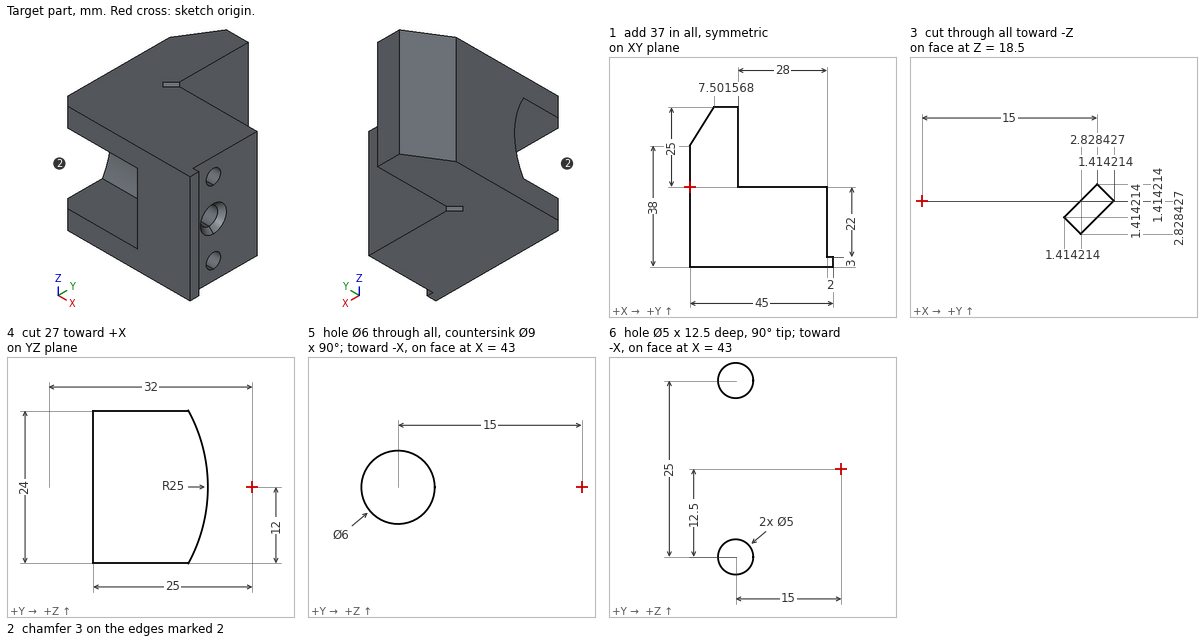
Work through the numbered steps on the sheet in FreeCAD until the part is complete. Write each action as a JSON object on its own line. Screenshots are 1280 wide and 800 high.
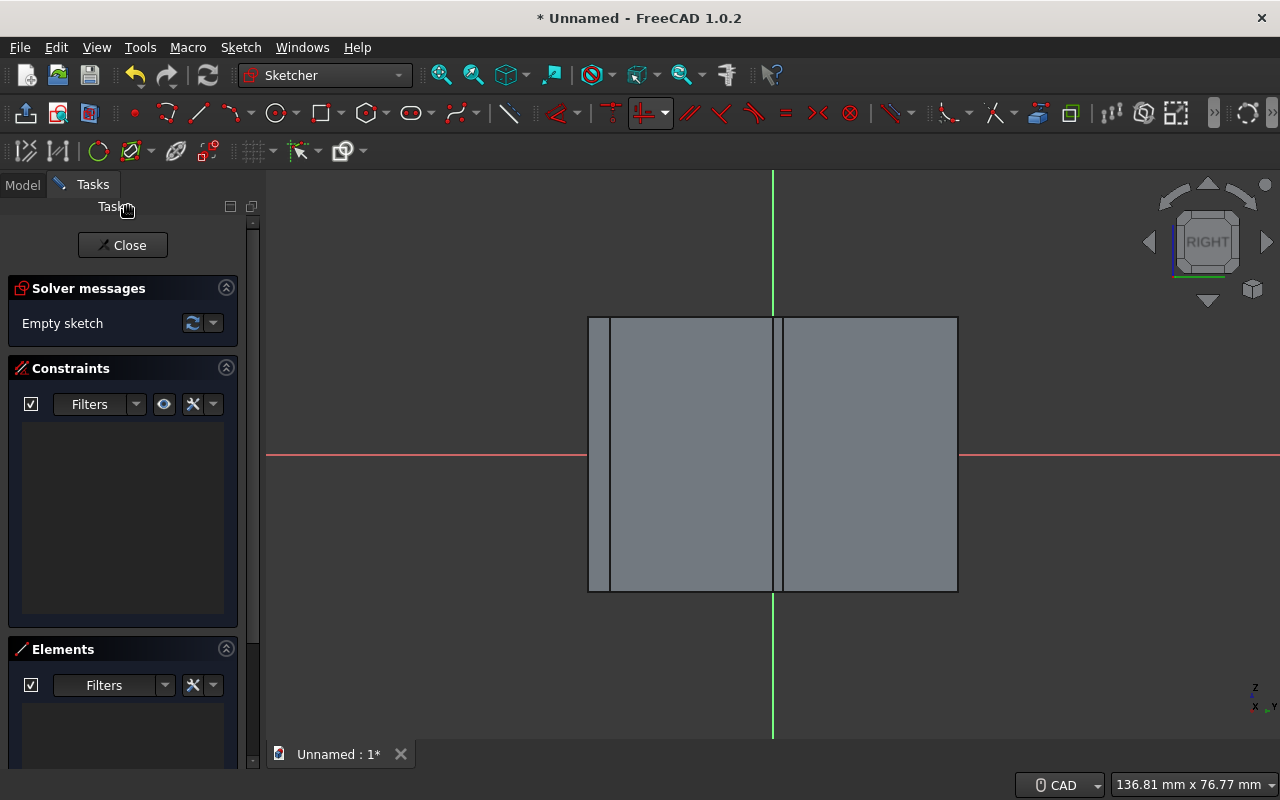
{"action": "left_click", "coordinate": [90, 114]}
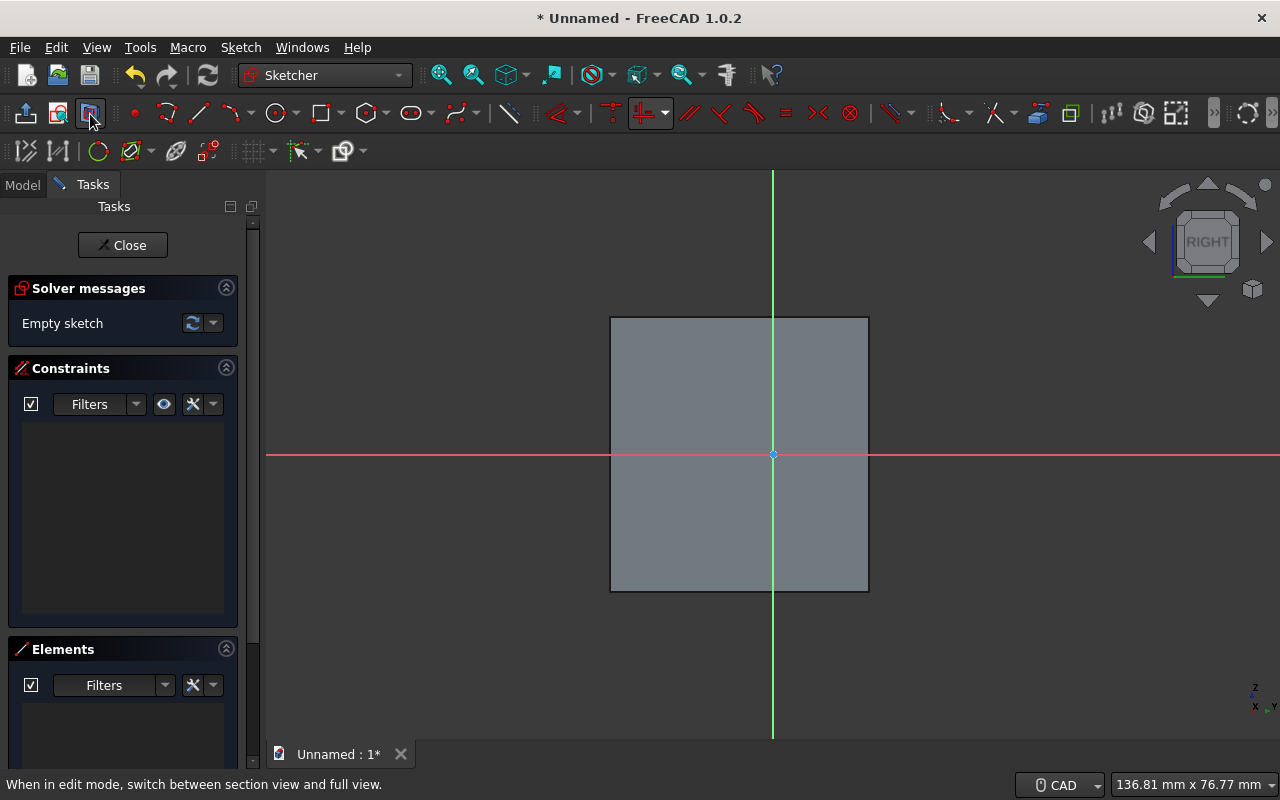
{"action": "scroll", "coordinate": [661, 454], "scroll_direction": "up", "scroll_amount": 4}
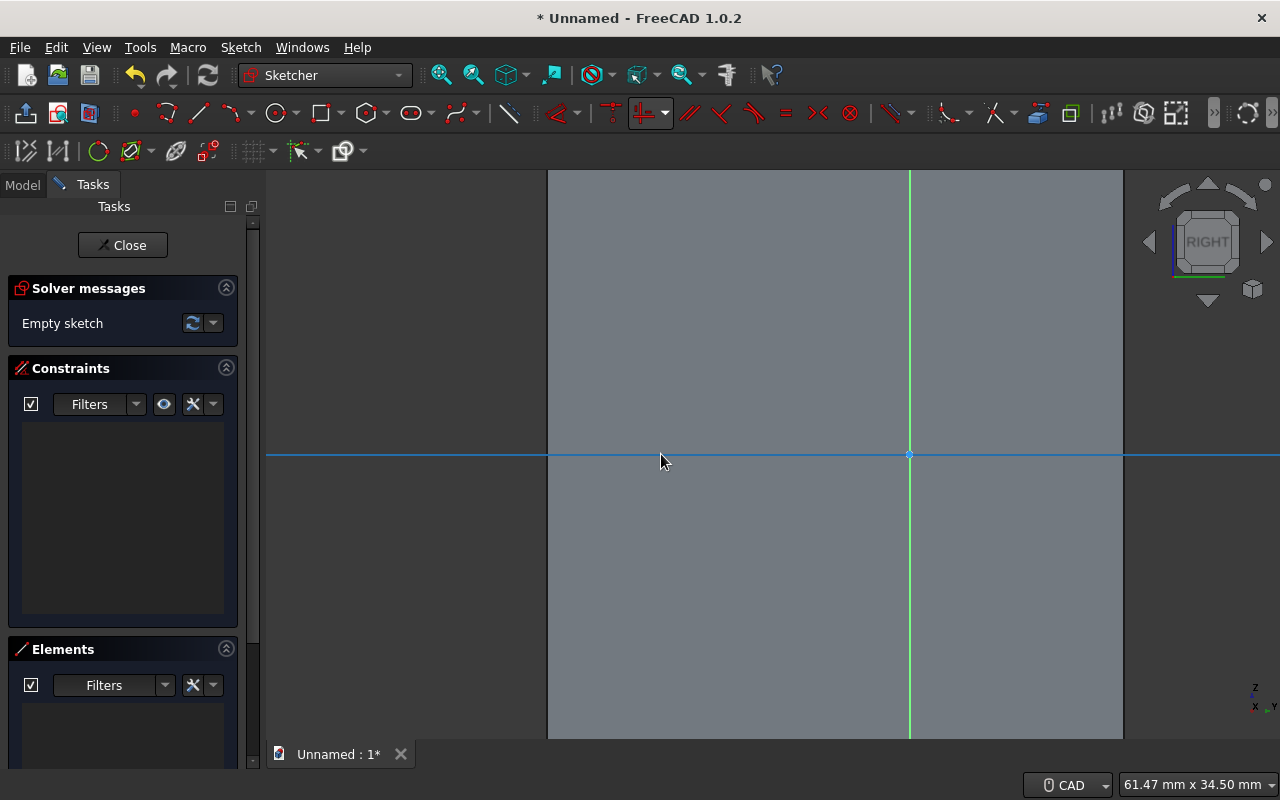
{"action": "left_click", "coordinate": [168, 114]}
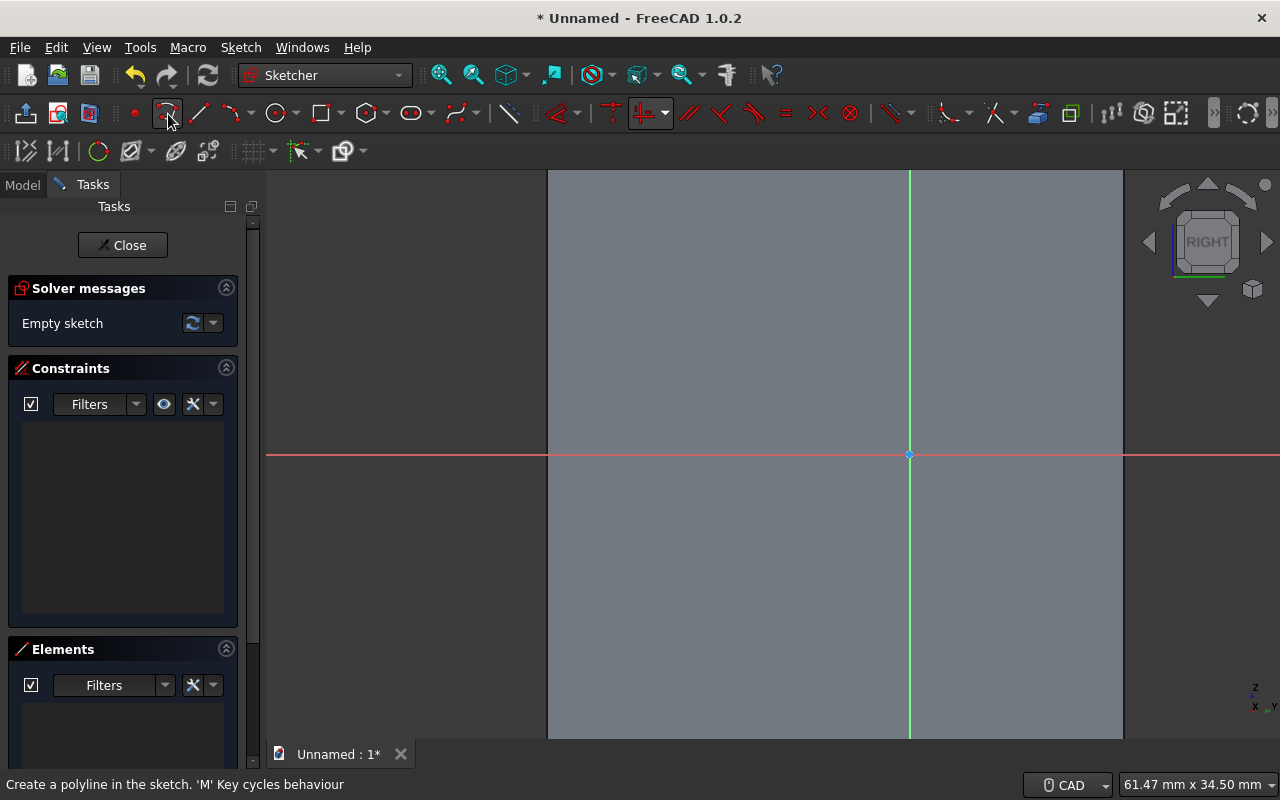
{"action": "left_click", "coordinate": [744, 652]}
{"action": "left_click", "coordinate": [497, 652]}
{"action": "left_click", "coordinate": [497, 257]}
{"action": "left_click", "coordinate": [744, 257]}
{"action": "right_click", "coordinate": [744, 257]}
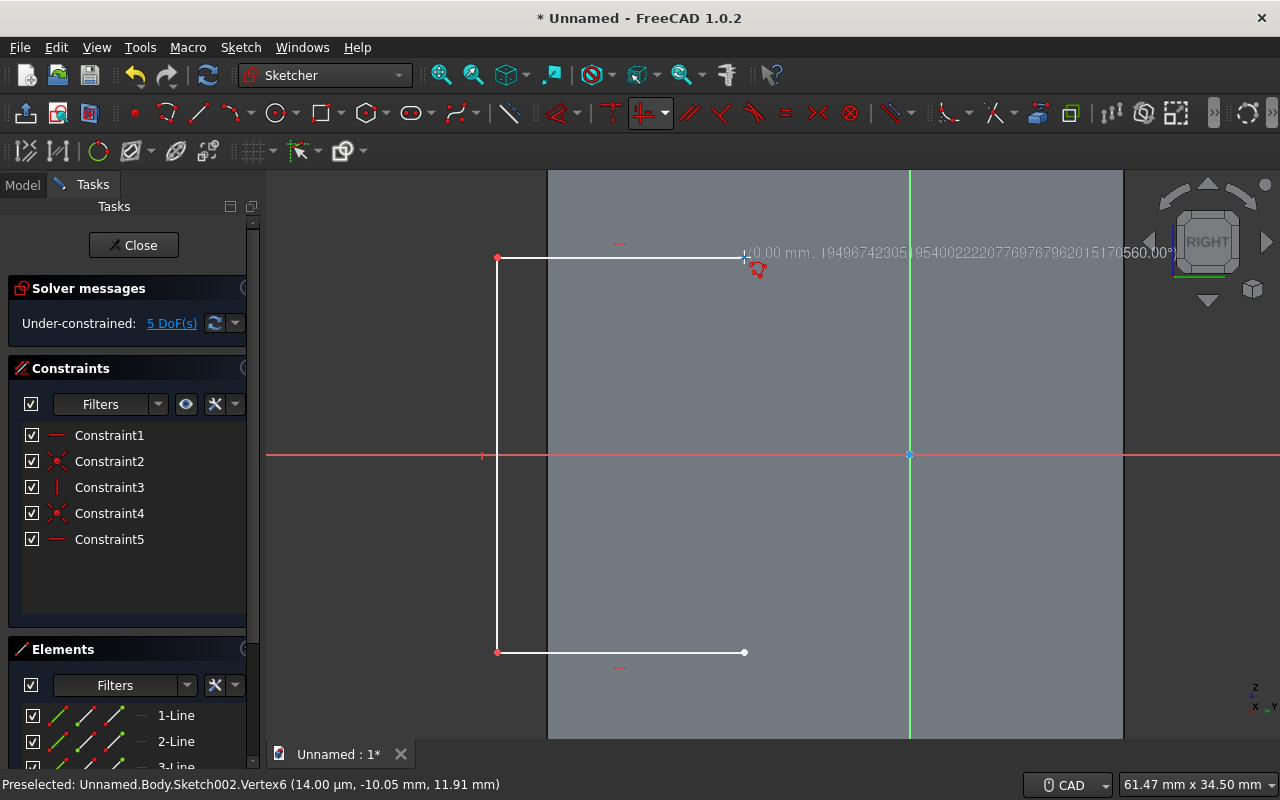
{"action": "left_click", "coordinate": [232, 114]}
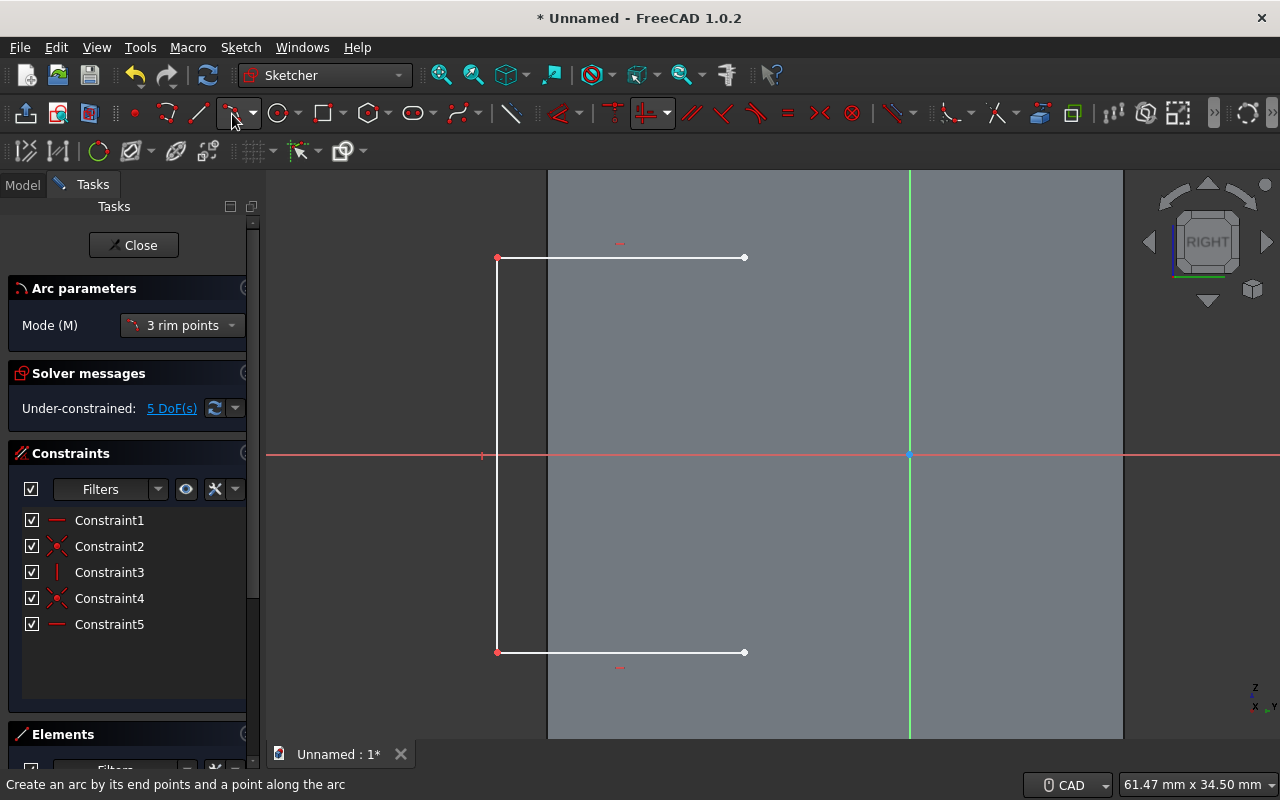
{"action": "left_click", "coordinate": [744, 258]}
{"action": "left_click", "coordinate": [744, 653]}
{"action": "left_click", "coordinate": [792, 496]}
{"action": "key", "text": "Escape"}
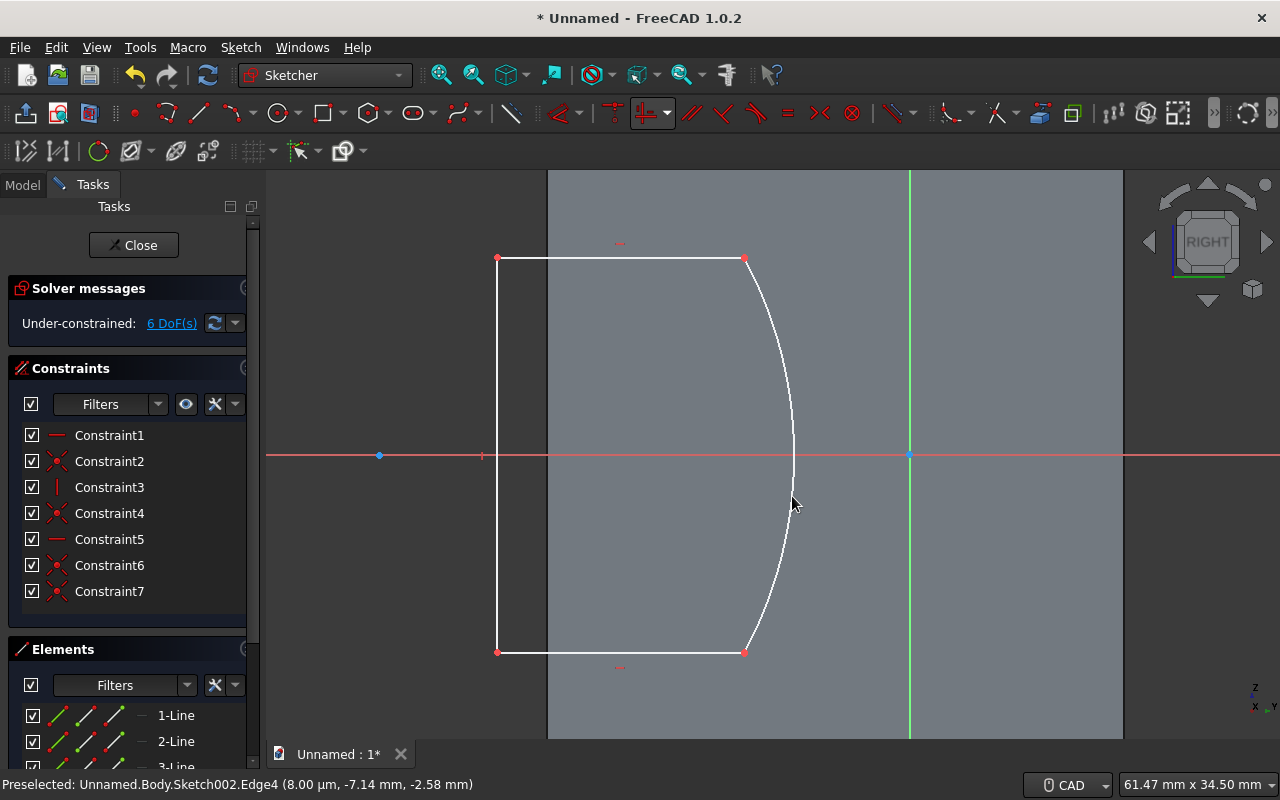
{"action": "left_click", "coordinate": [380, 456]}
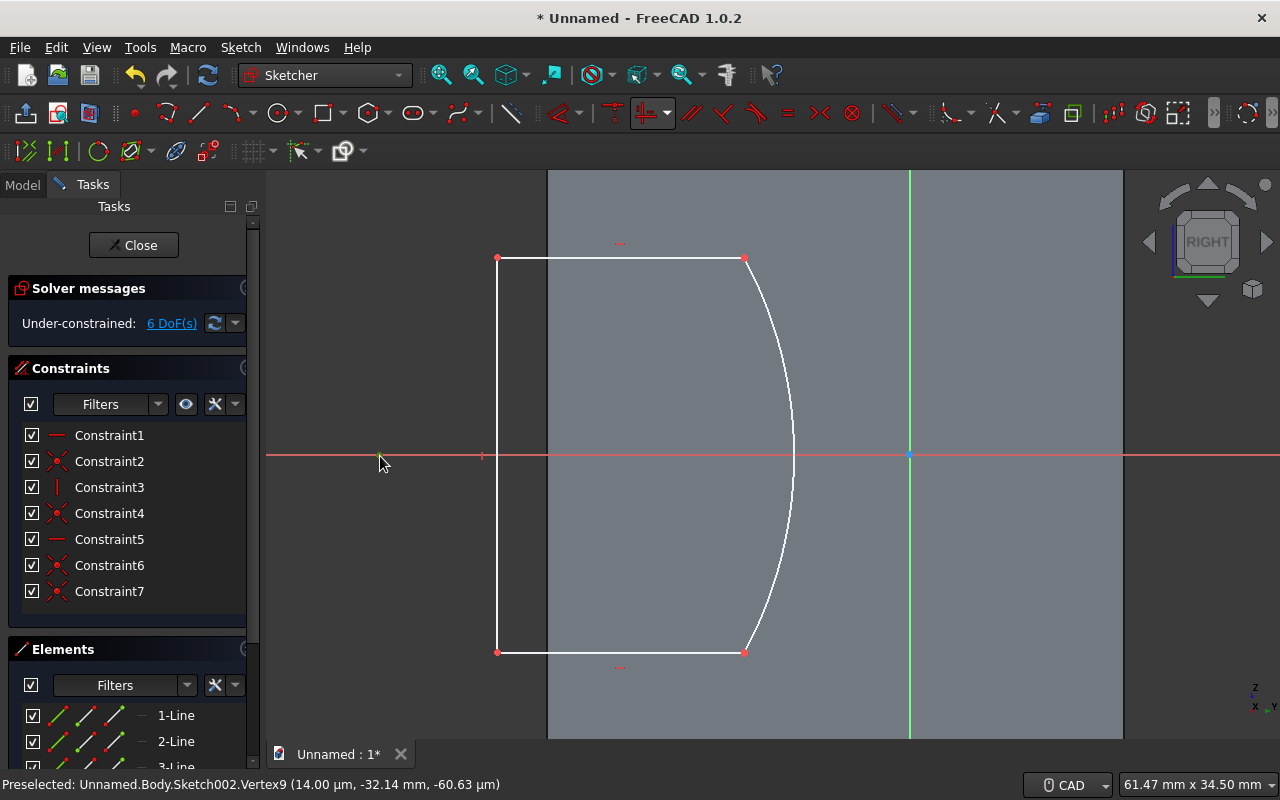
{"action": "left_click", "coordinate": [353, 454]}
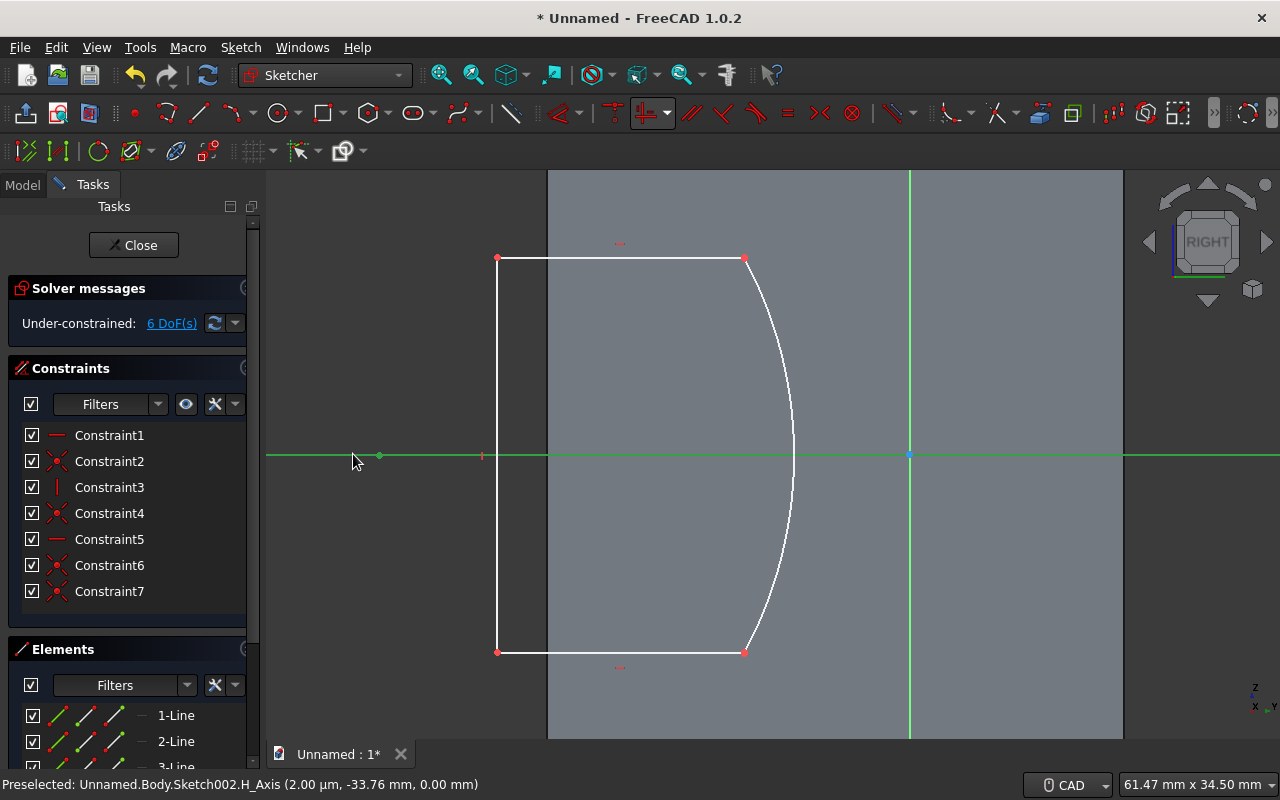
{"action": "left_click", "coordinate": [614, 114]}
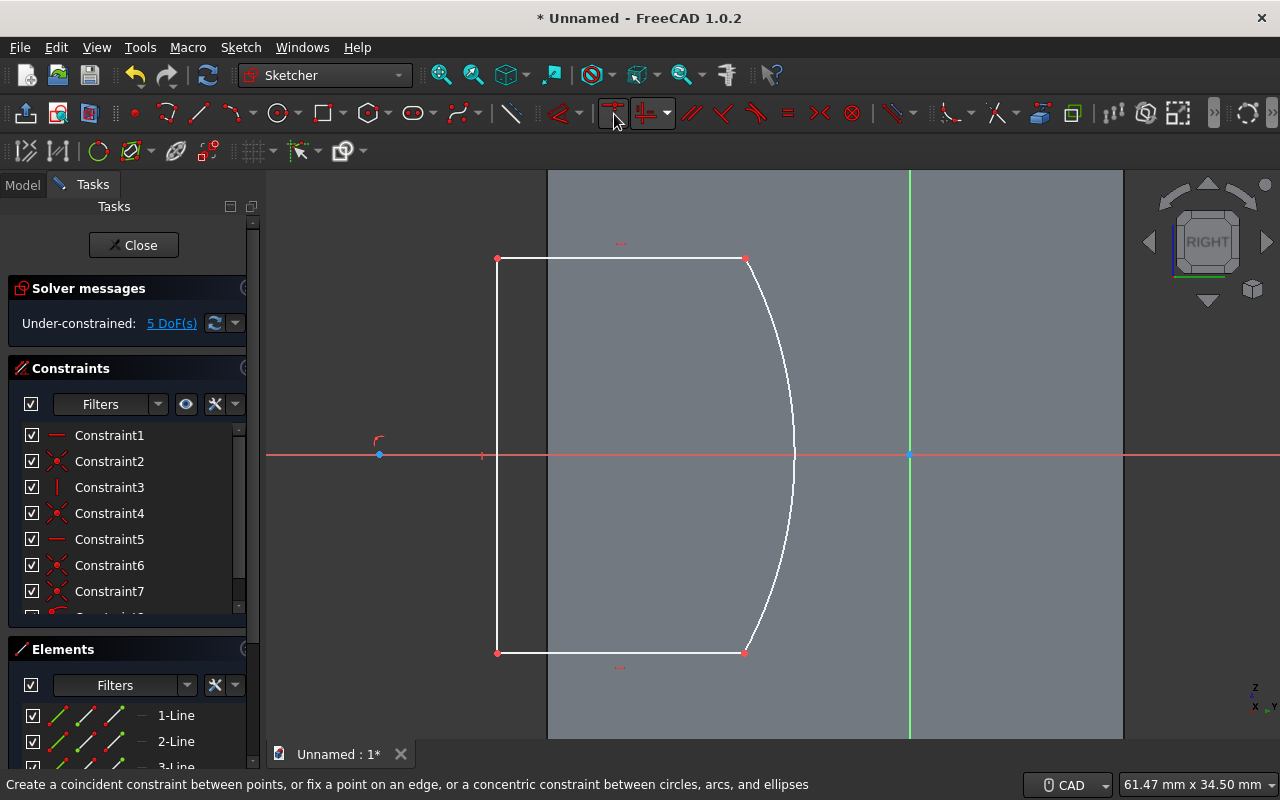
{"action": "left_click", "coordinate": [558, 114]}